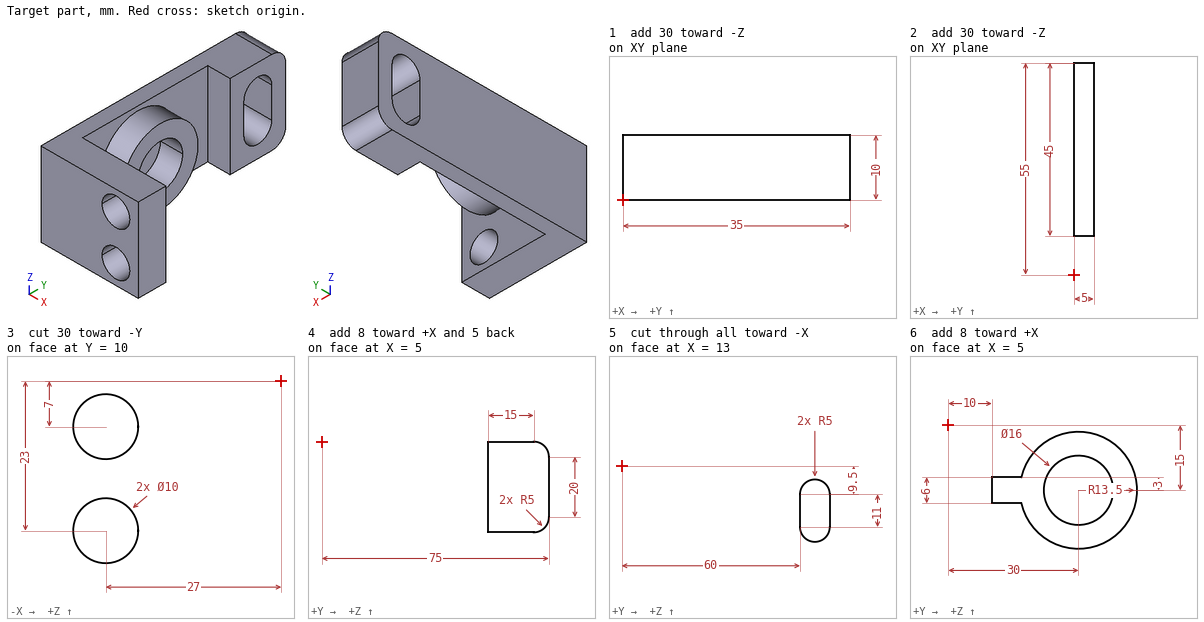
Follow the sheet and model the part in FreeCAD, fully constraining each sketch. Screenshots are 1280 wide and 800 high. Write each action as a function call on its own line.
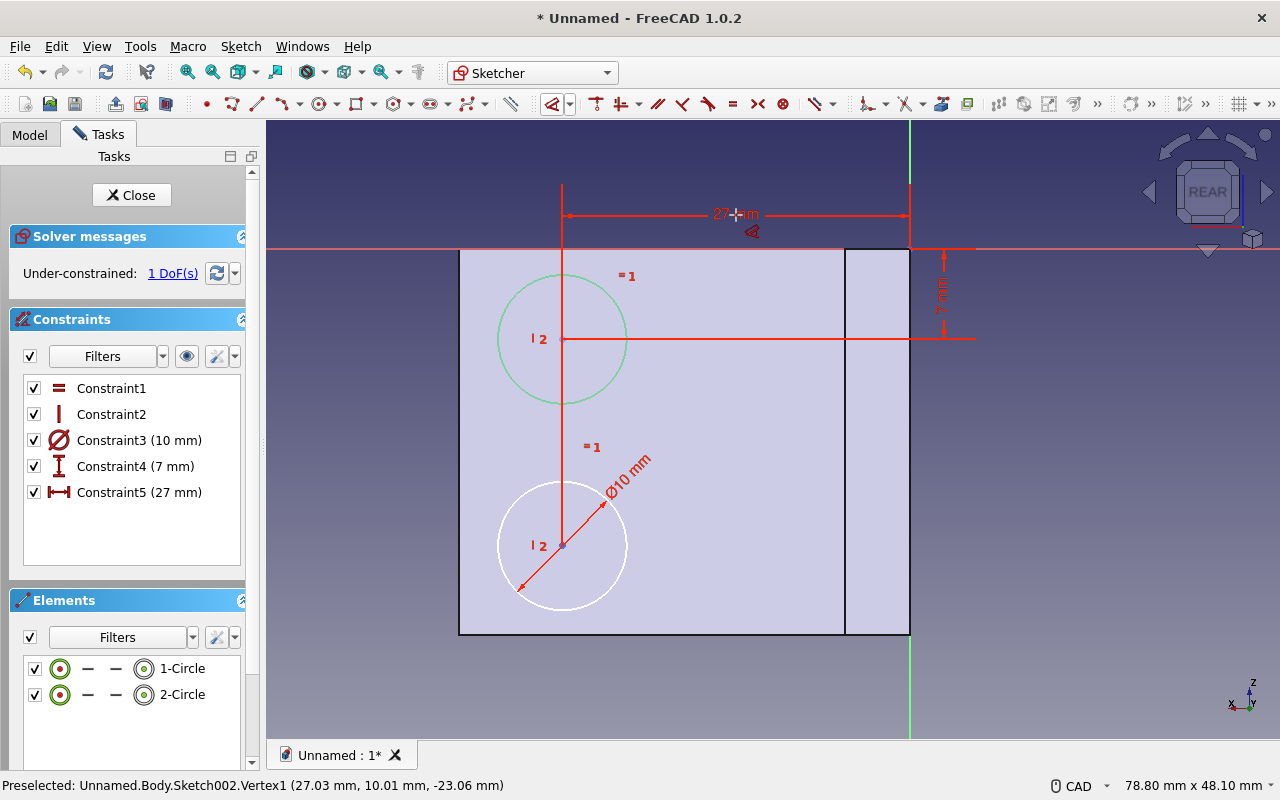
click(562, 546)
click(944, 398)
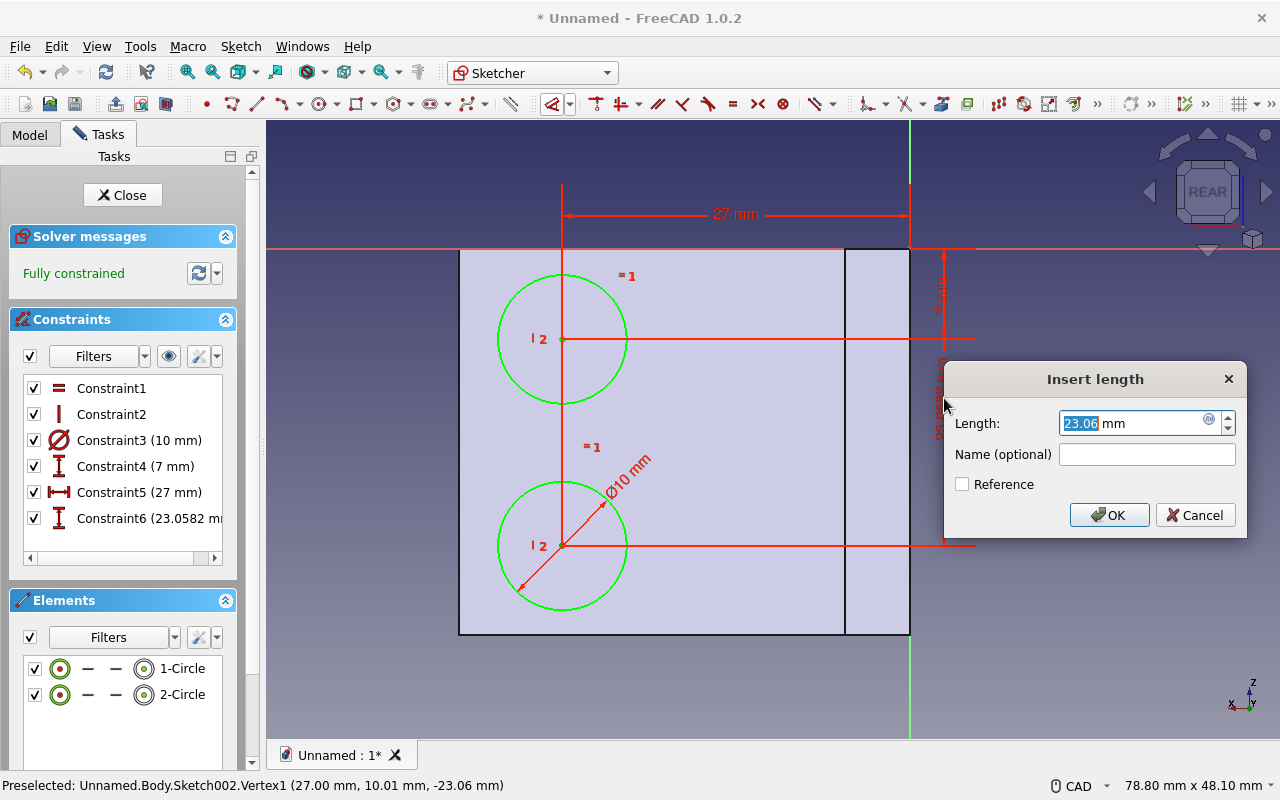
text(23)
key(Return)
key(Escape)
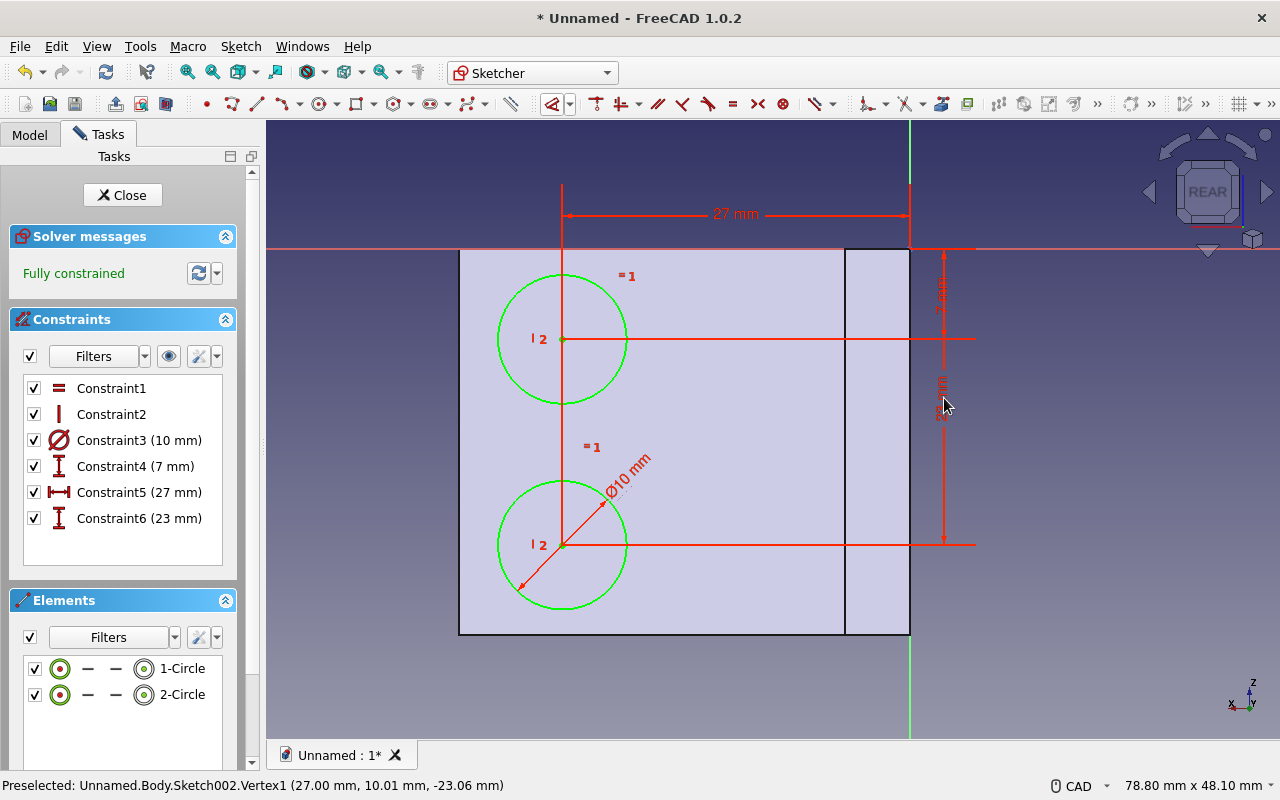
click(123, 195)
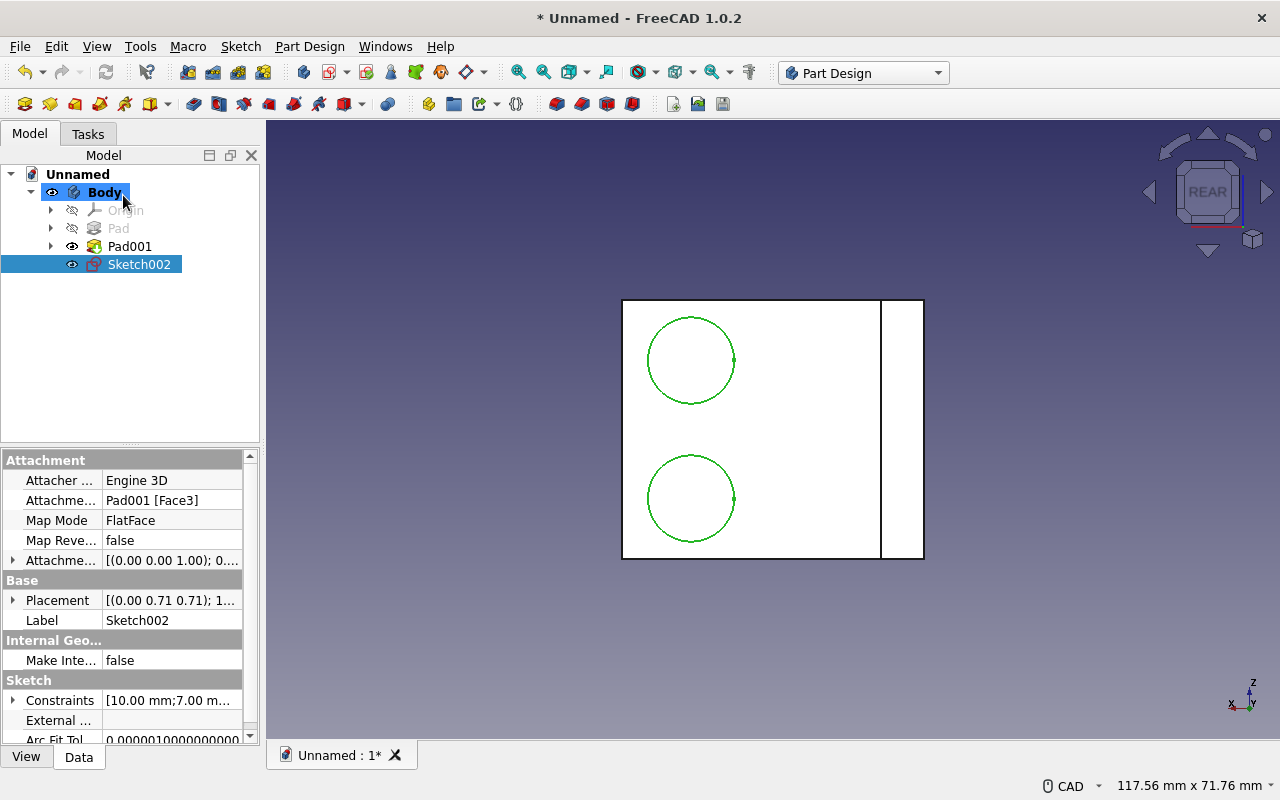
click(194, 104)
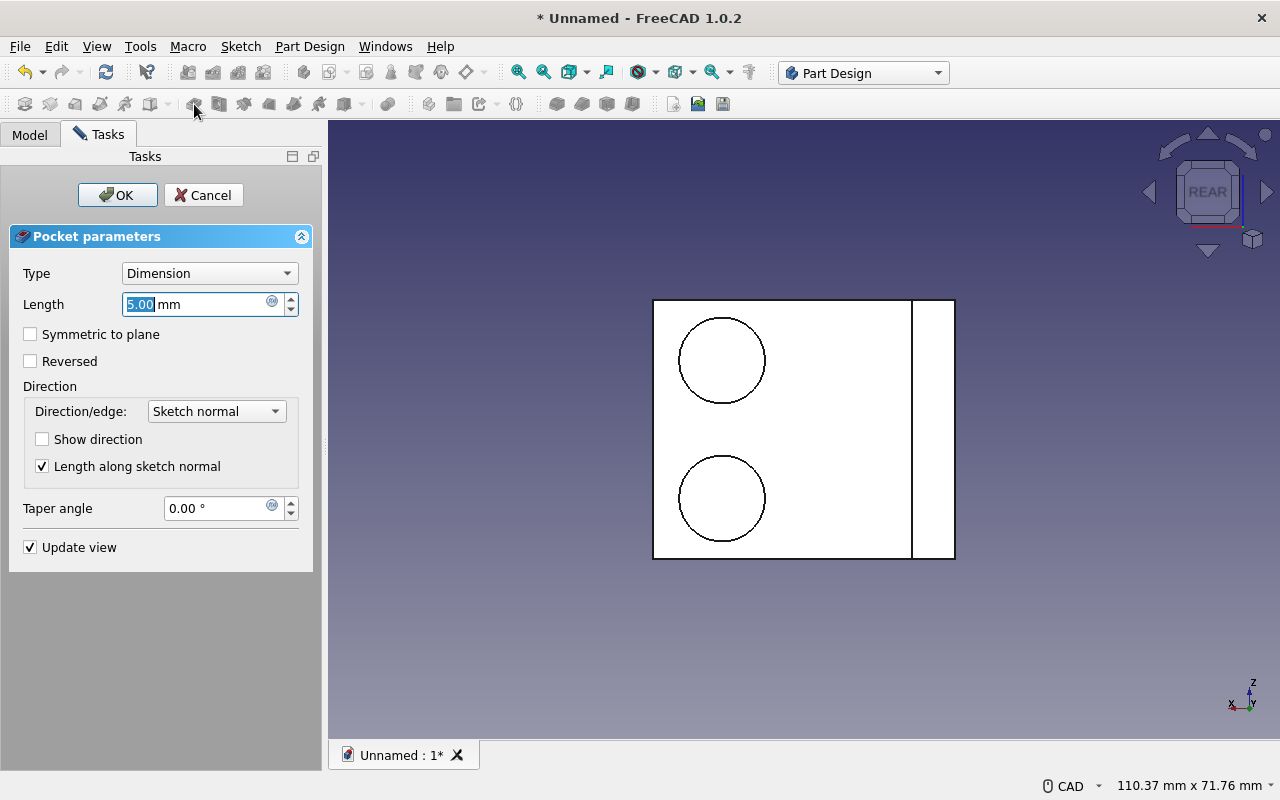
text(30)
key(Tab)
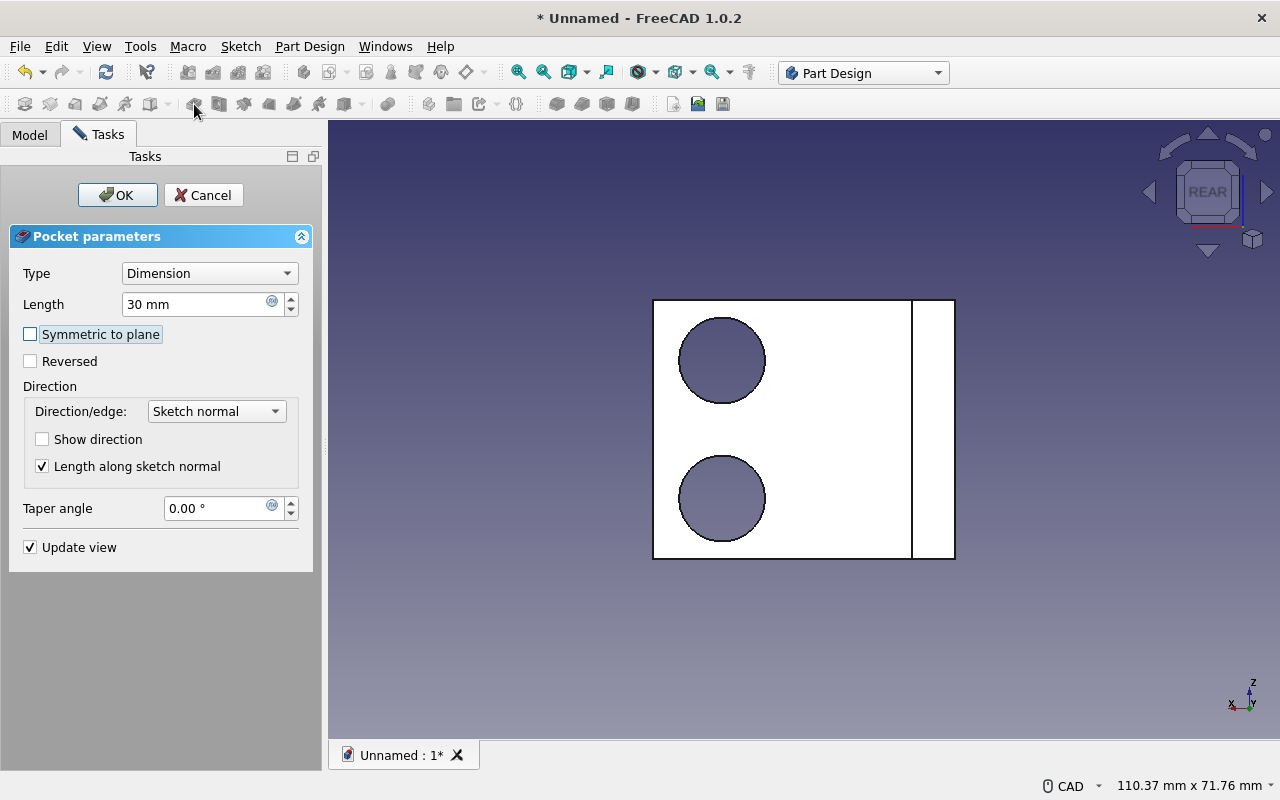
click(118, 195)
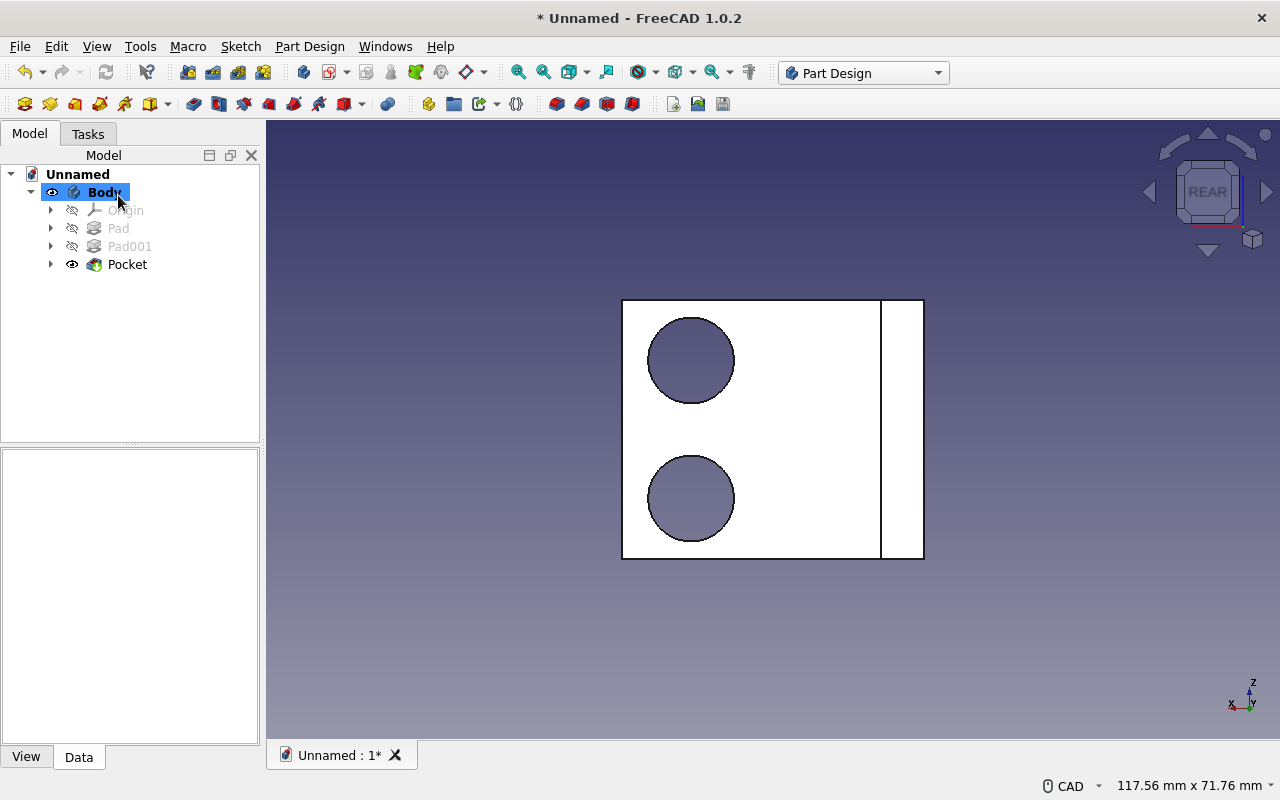
key(v)
key(f)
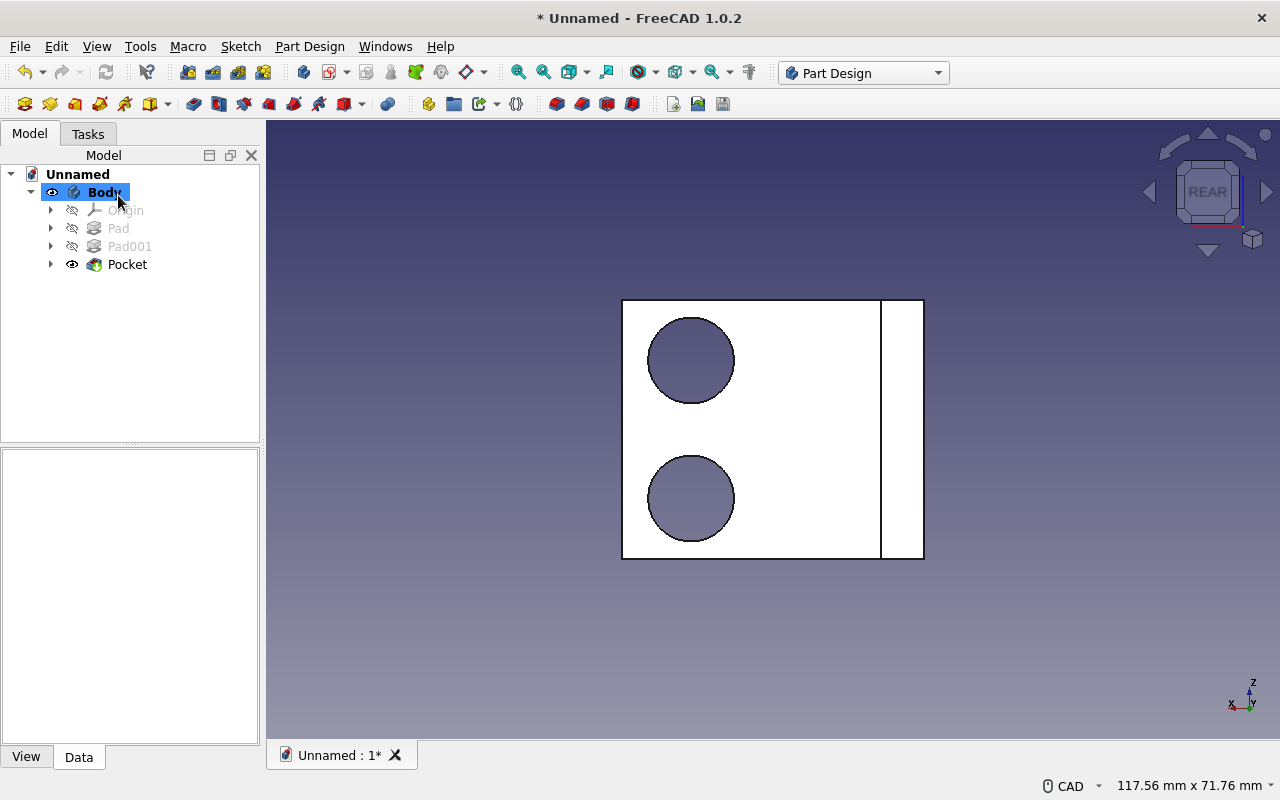
key(0)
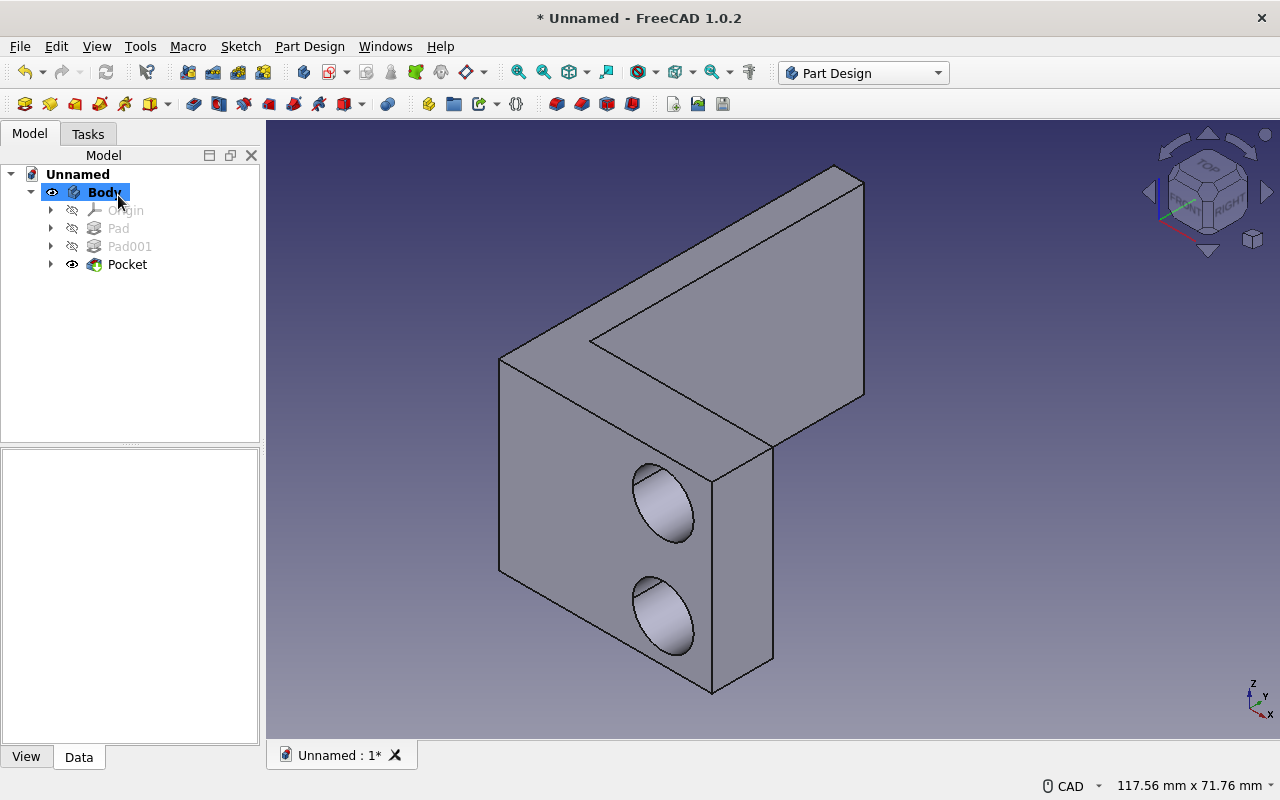
click(766, 344)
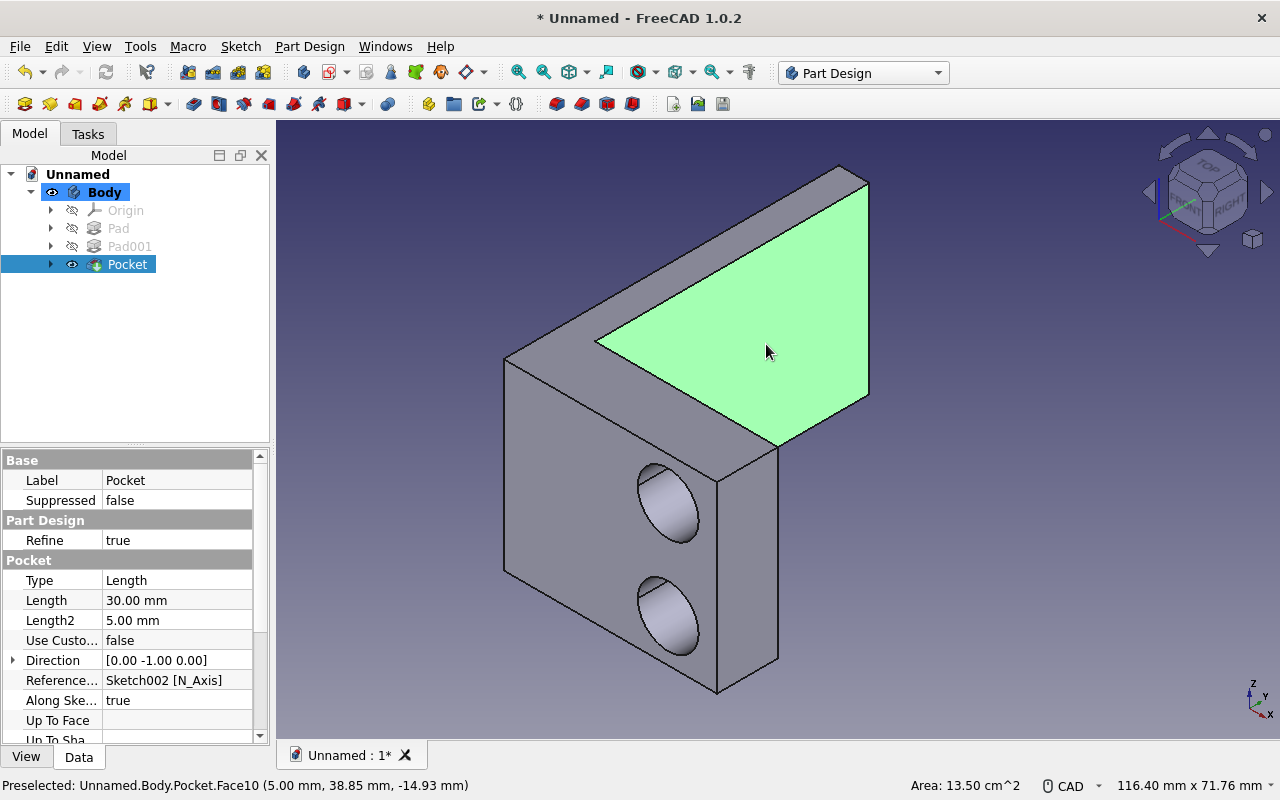
click(328, 72)